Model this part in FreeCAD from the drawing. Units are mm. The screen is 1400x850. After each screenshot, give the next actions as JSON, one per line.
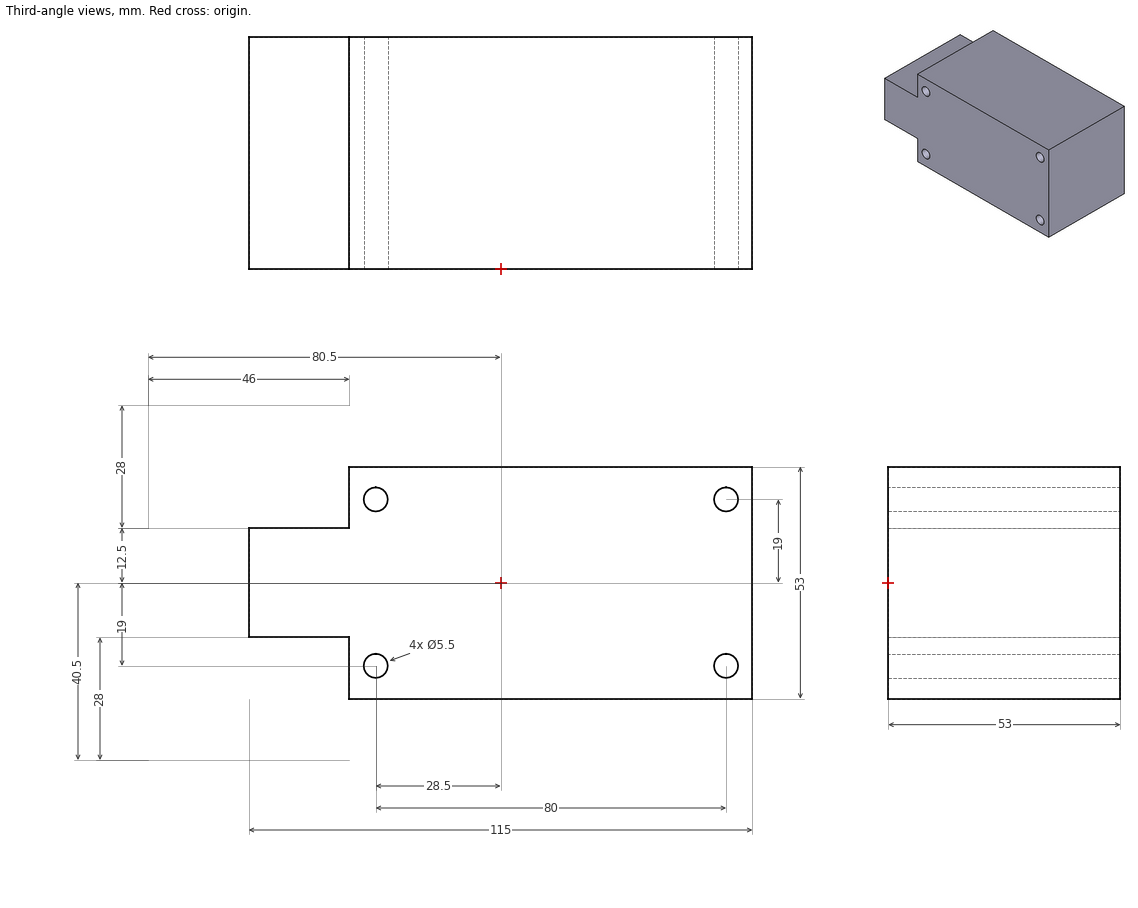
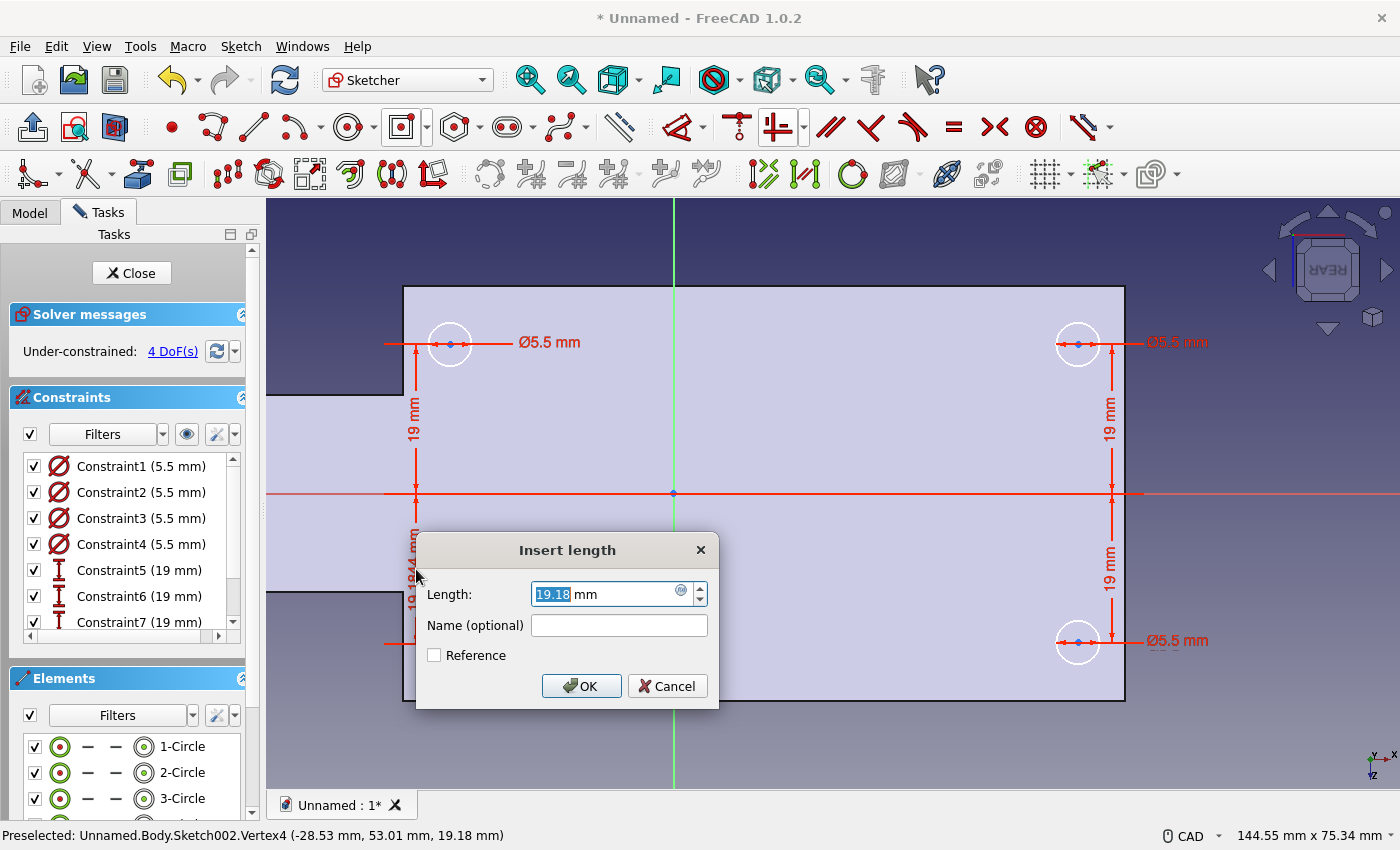
{"action": "type", "text": "19"}
{"action": "key", "text": "Return"}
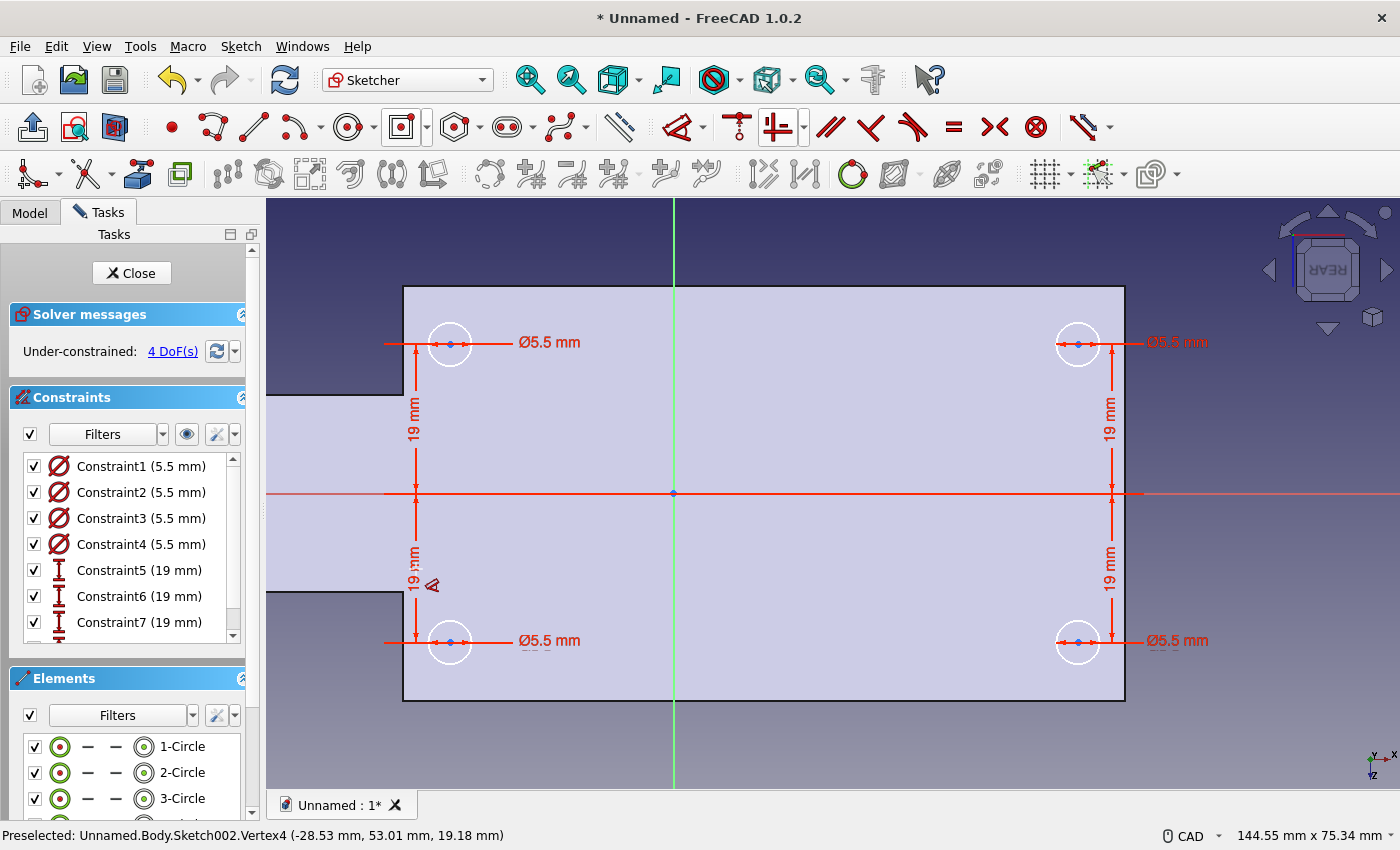
{"action": "left_click", "coordinate": [450, 344]}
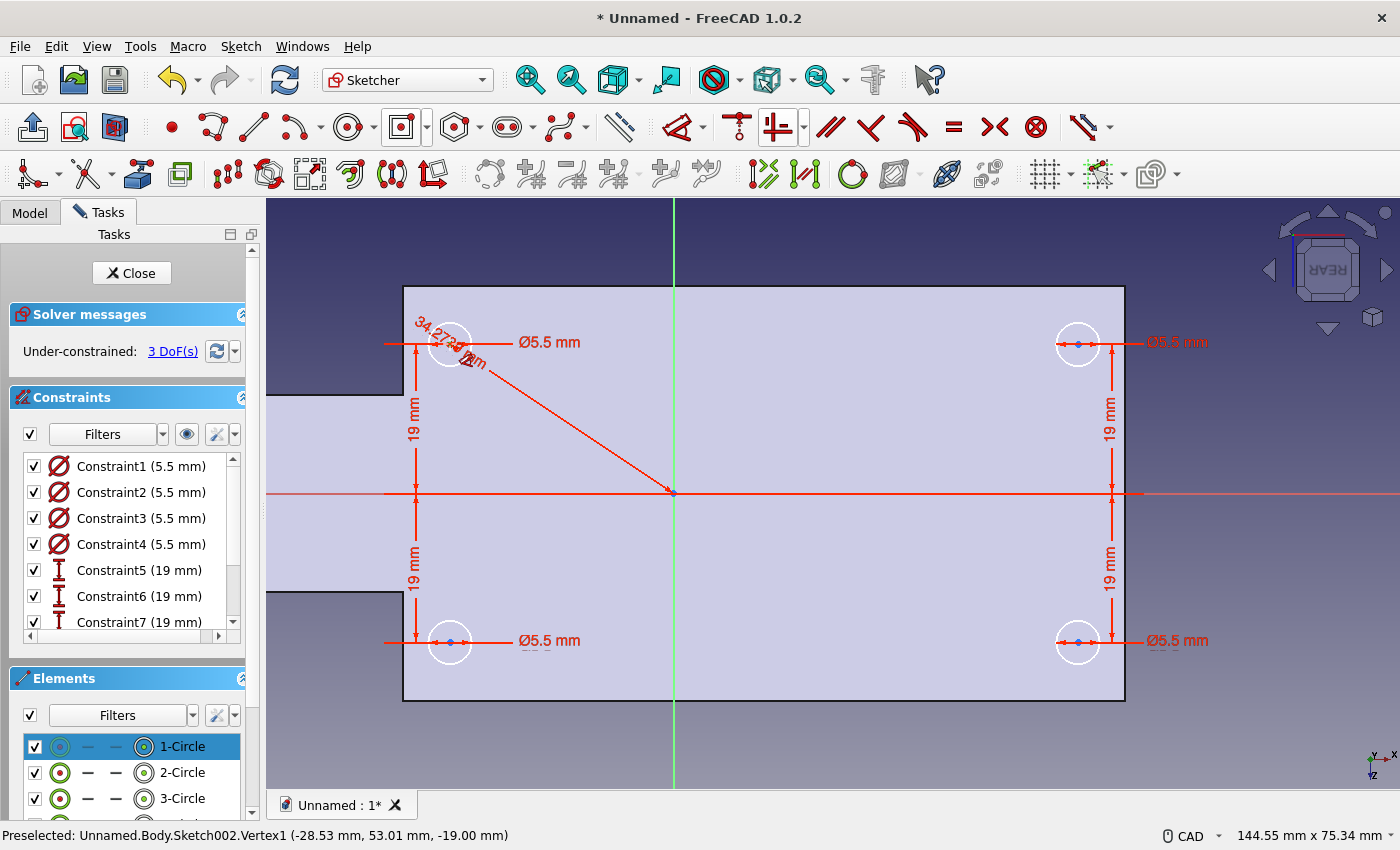
{"action": "left_click", "coordinate": [1078, 344]}
{"action": "left_click", "coordinate": [764, 310]}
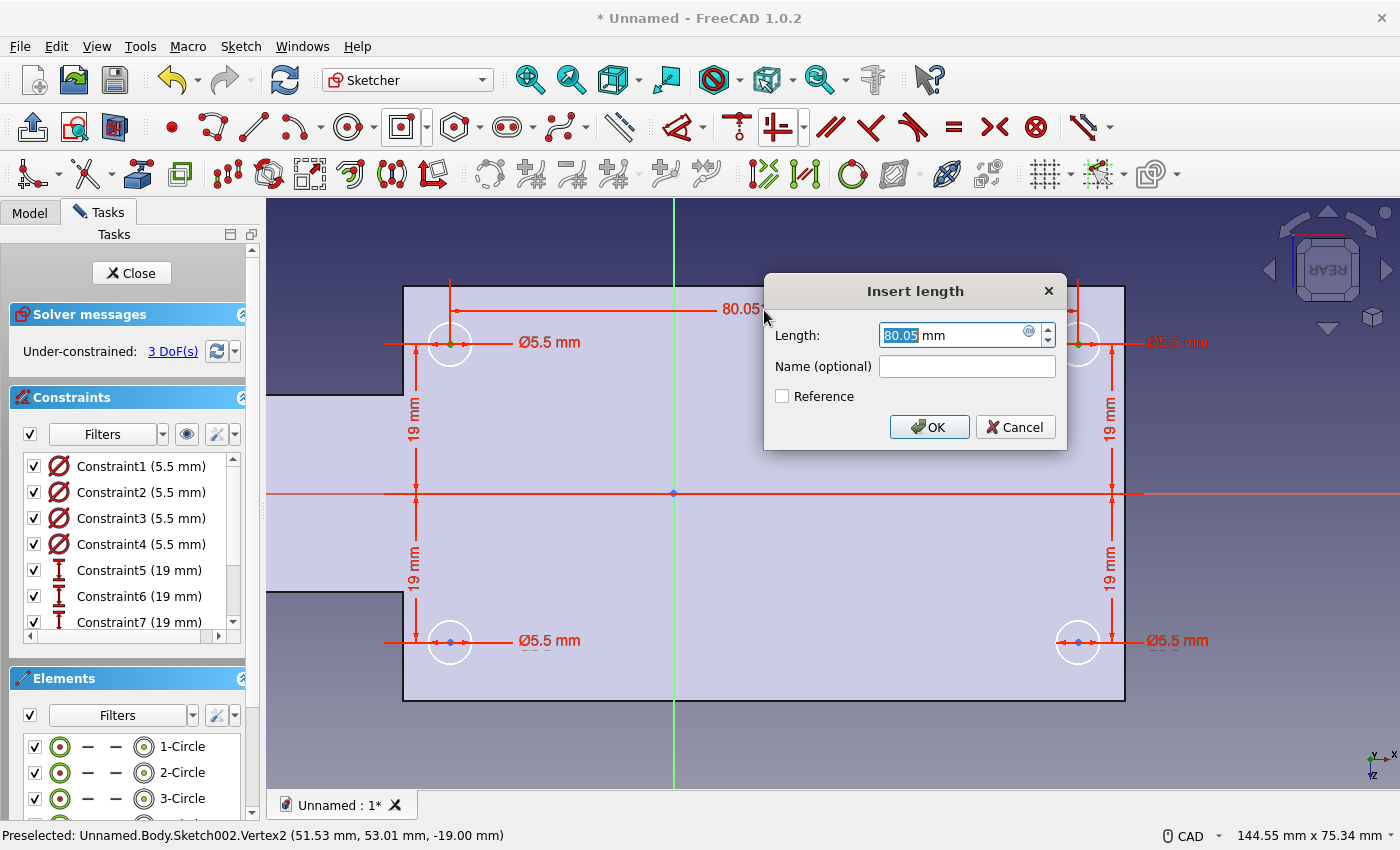
{"action": "type", "text": "80"}
{"action": "key", "text": "Return"}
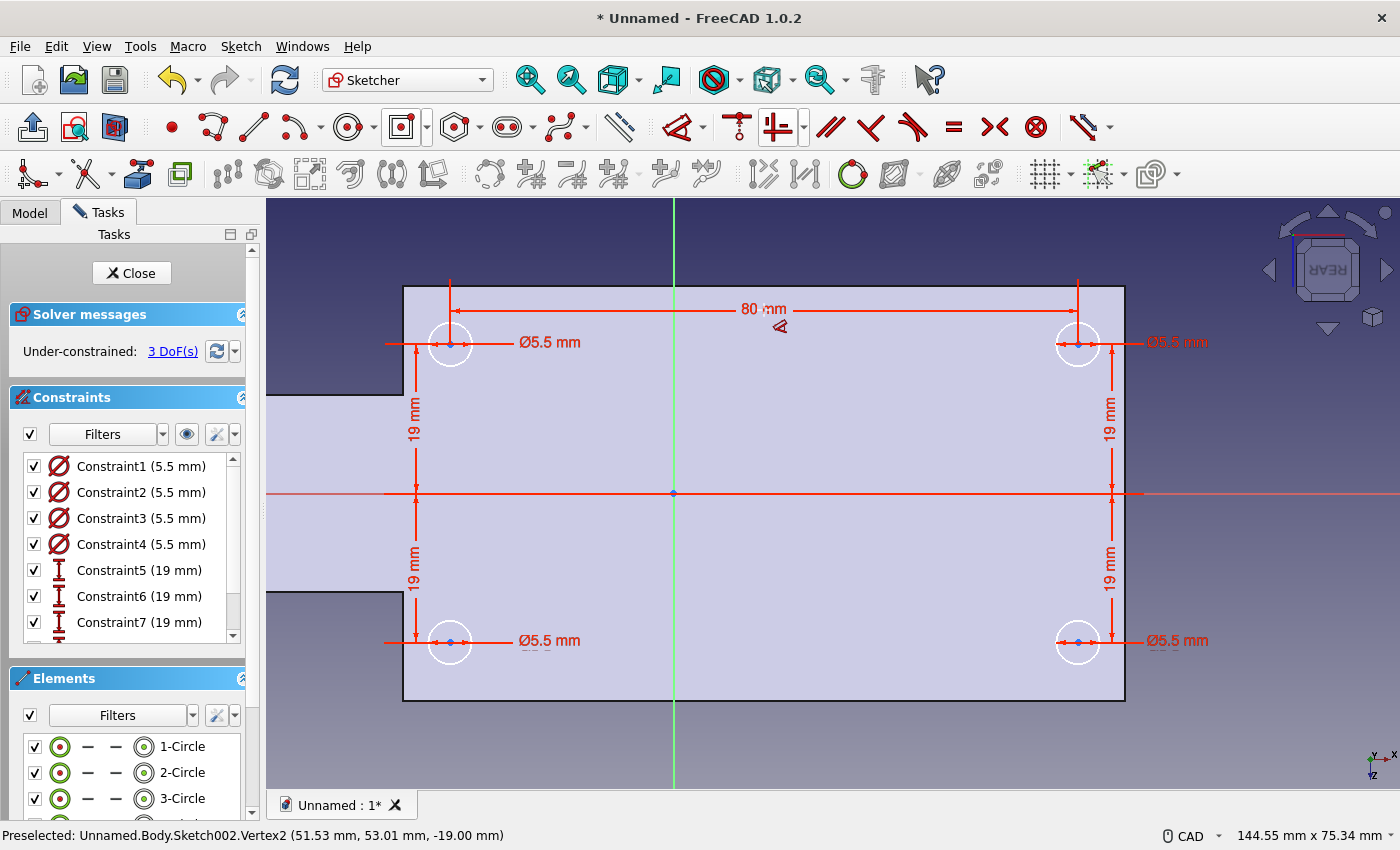
{"action": "left_click", "coordinate": [450, 344]}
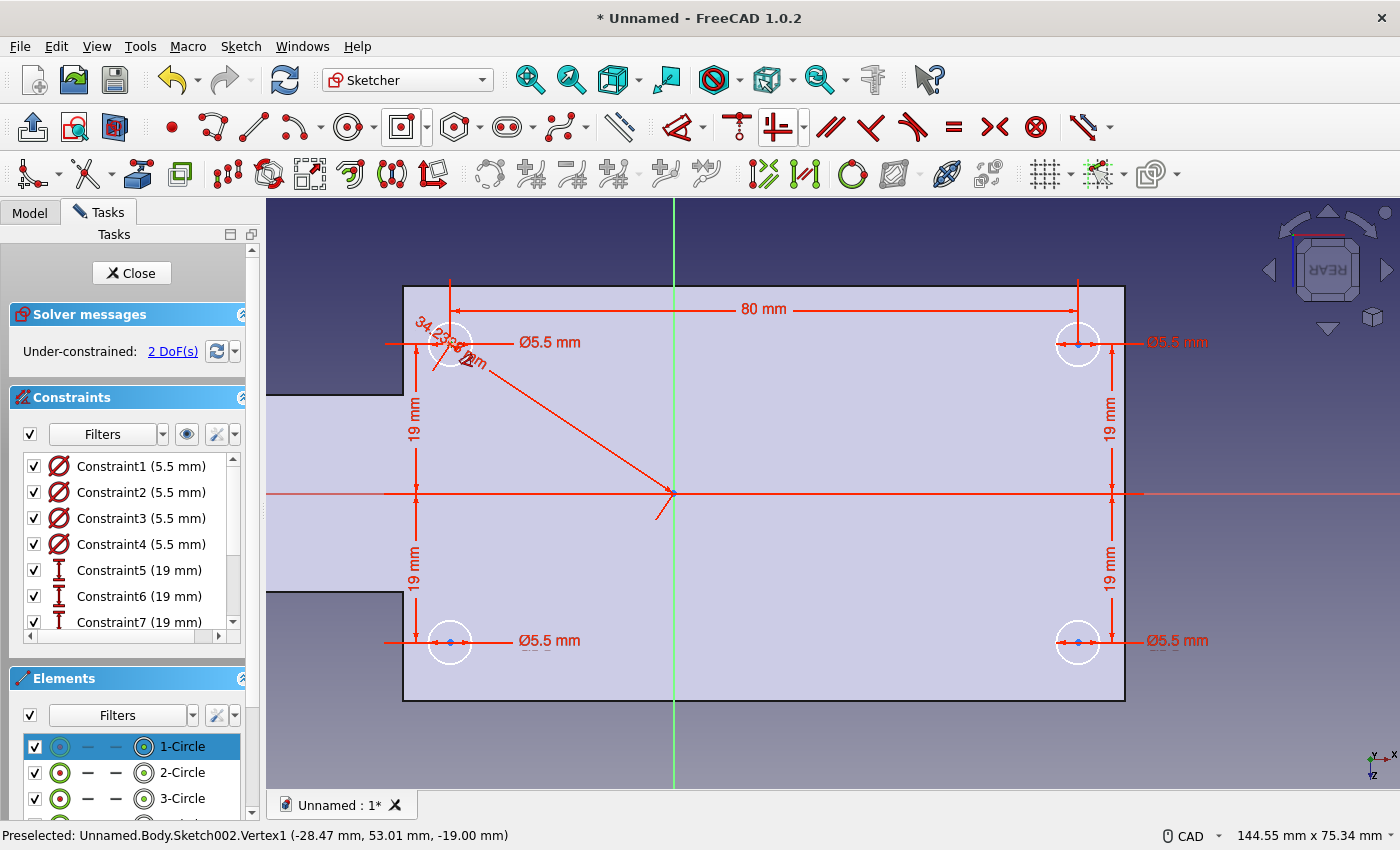
{"action": "left_click", "coordinate": [1078, 643]}
{"action": "left_click", "coordinate": [764, 677]}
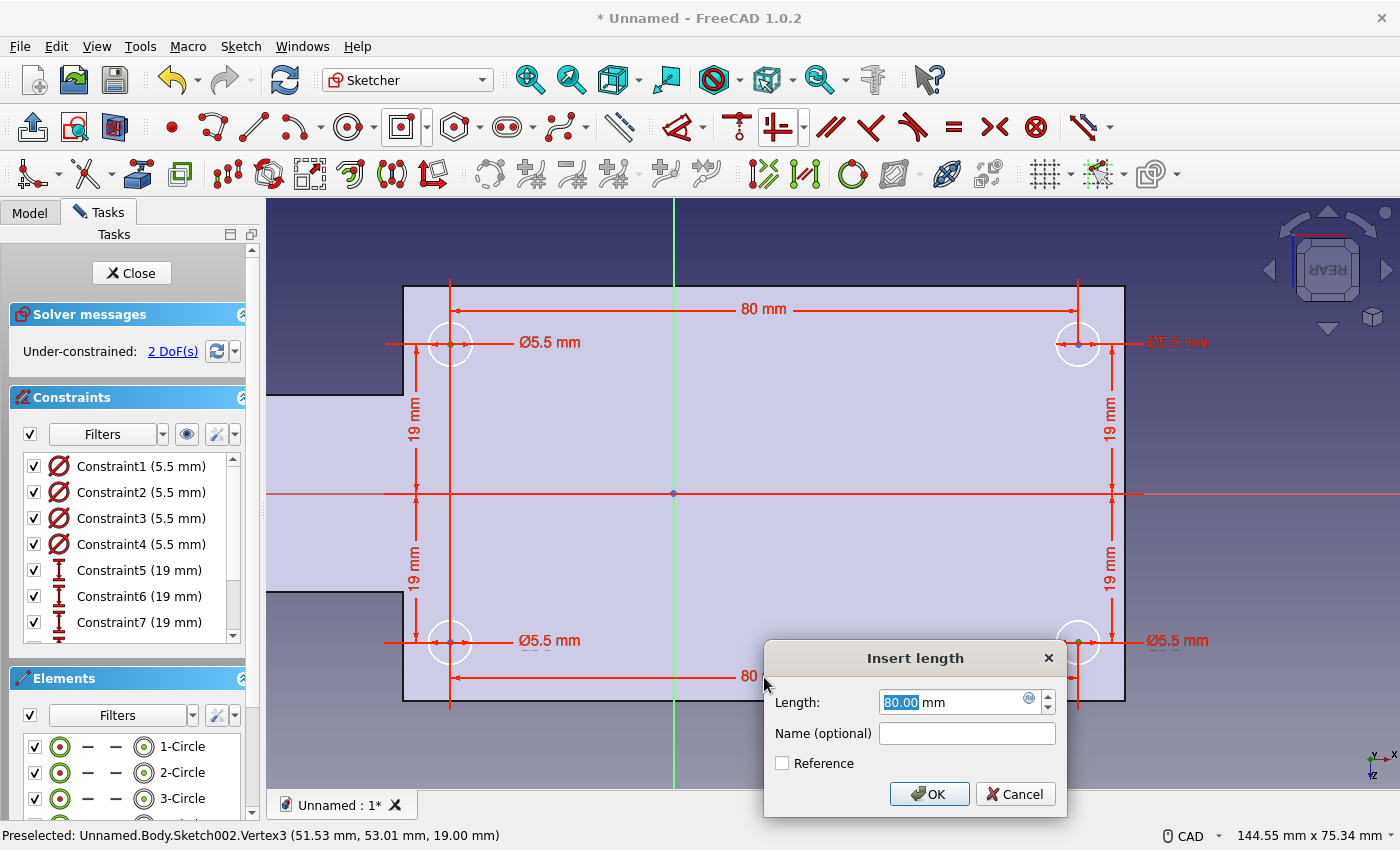
{"action": "type", "text": "80"}
{"action": "key", "text": "Return"}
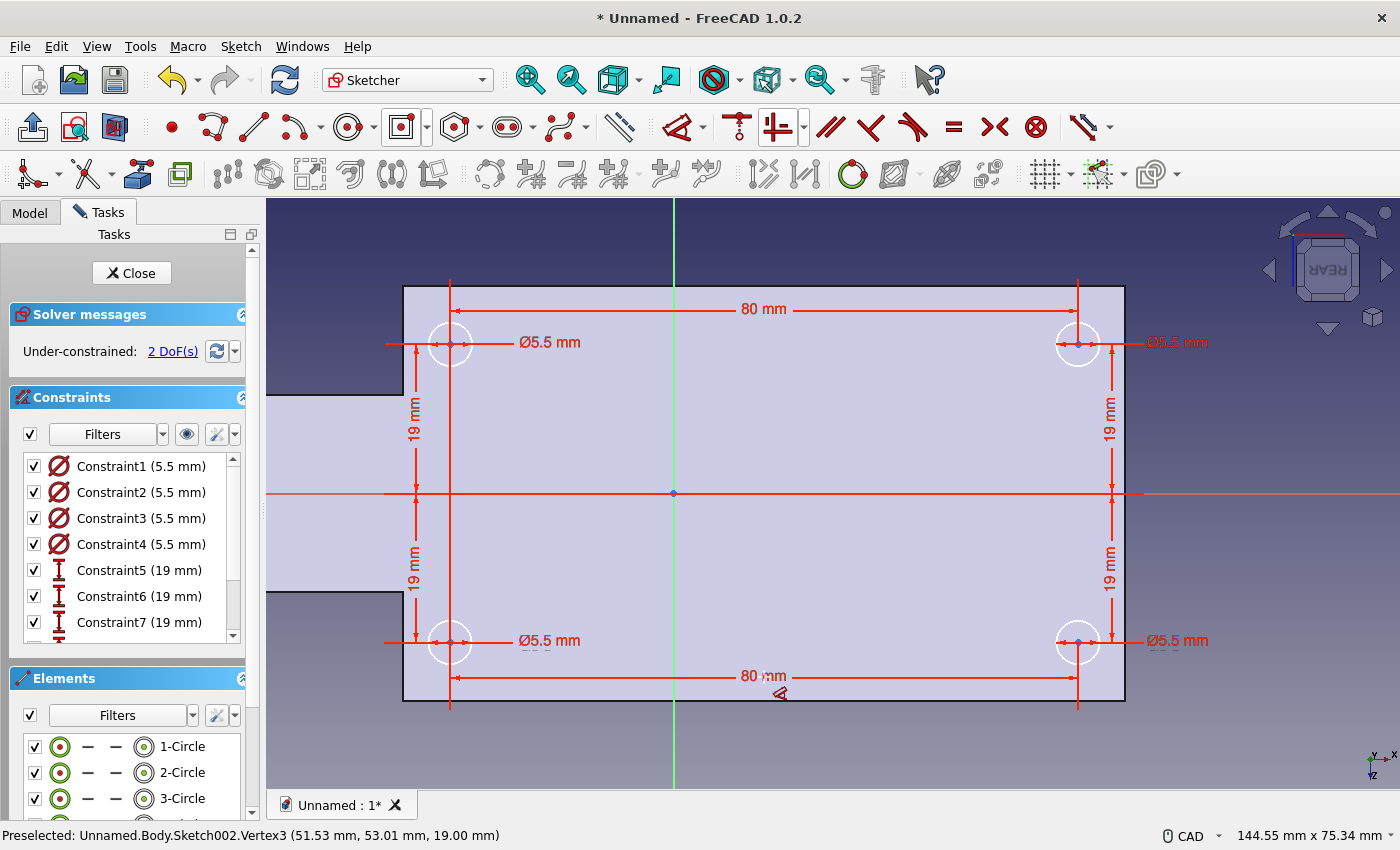
{"action": "left_click", "coordinate": [1078, 643]}